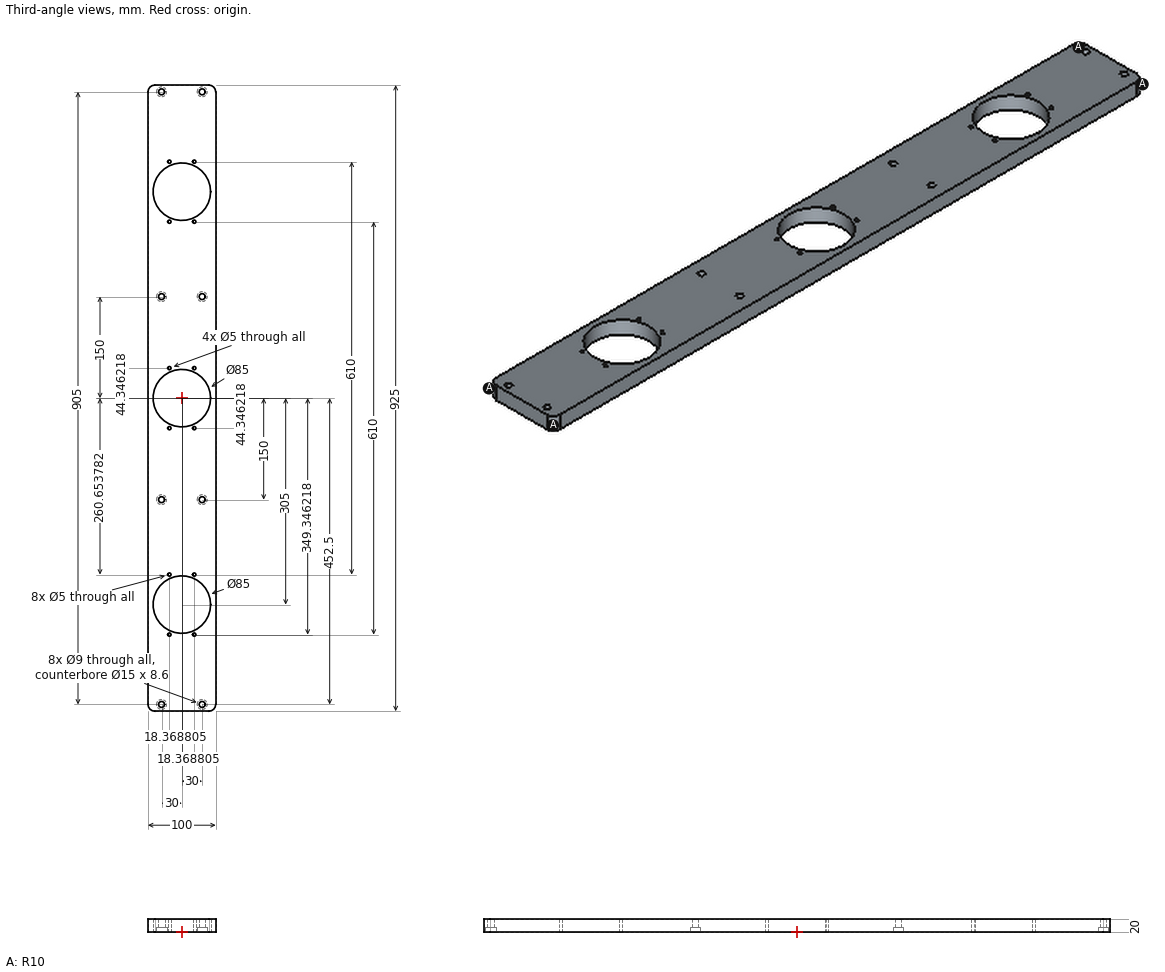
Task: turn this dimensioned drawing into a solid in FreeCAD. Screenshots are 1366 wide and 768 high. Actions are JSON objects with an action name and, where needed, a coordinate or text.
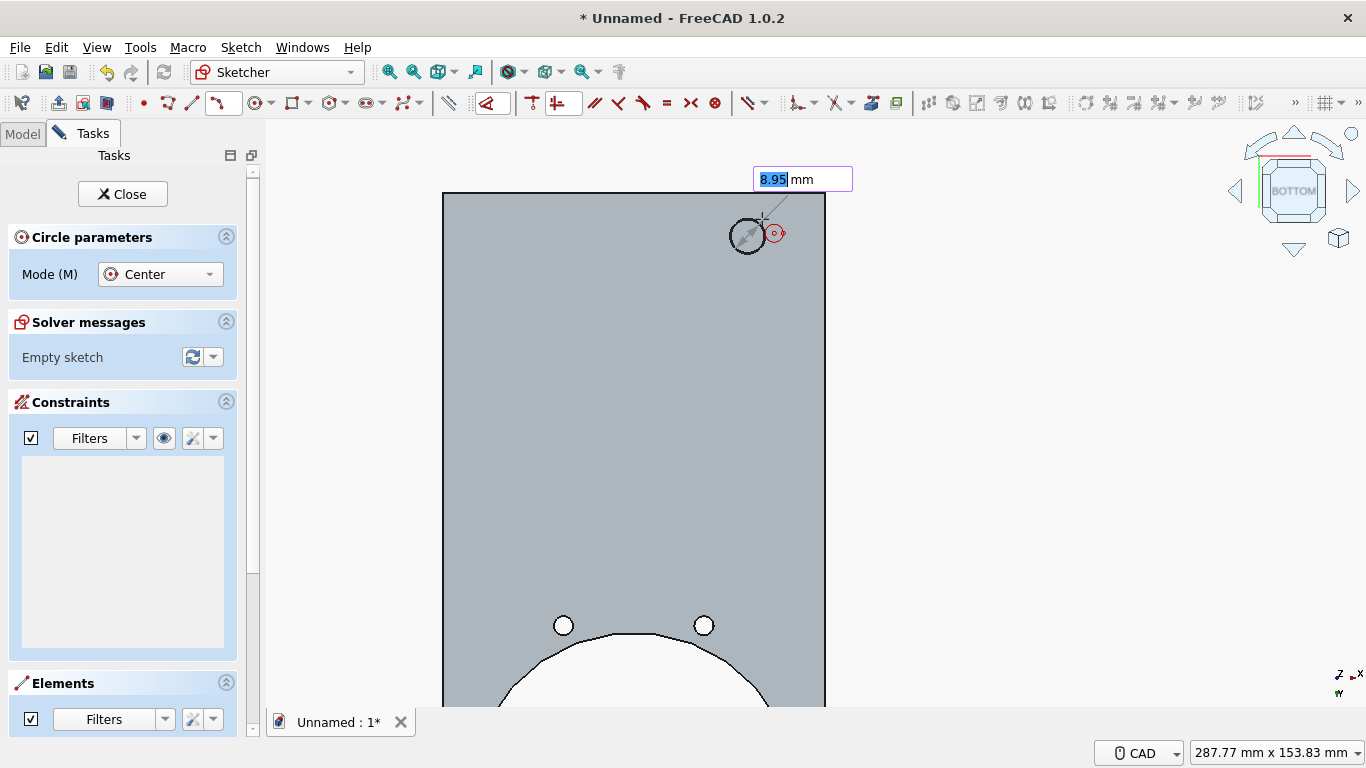
{"action": "left_click", "coordinate": [761, 219]}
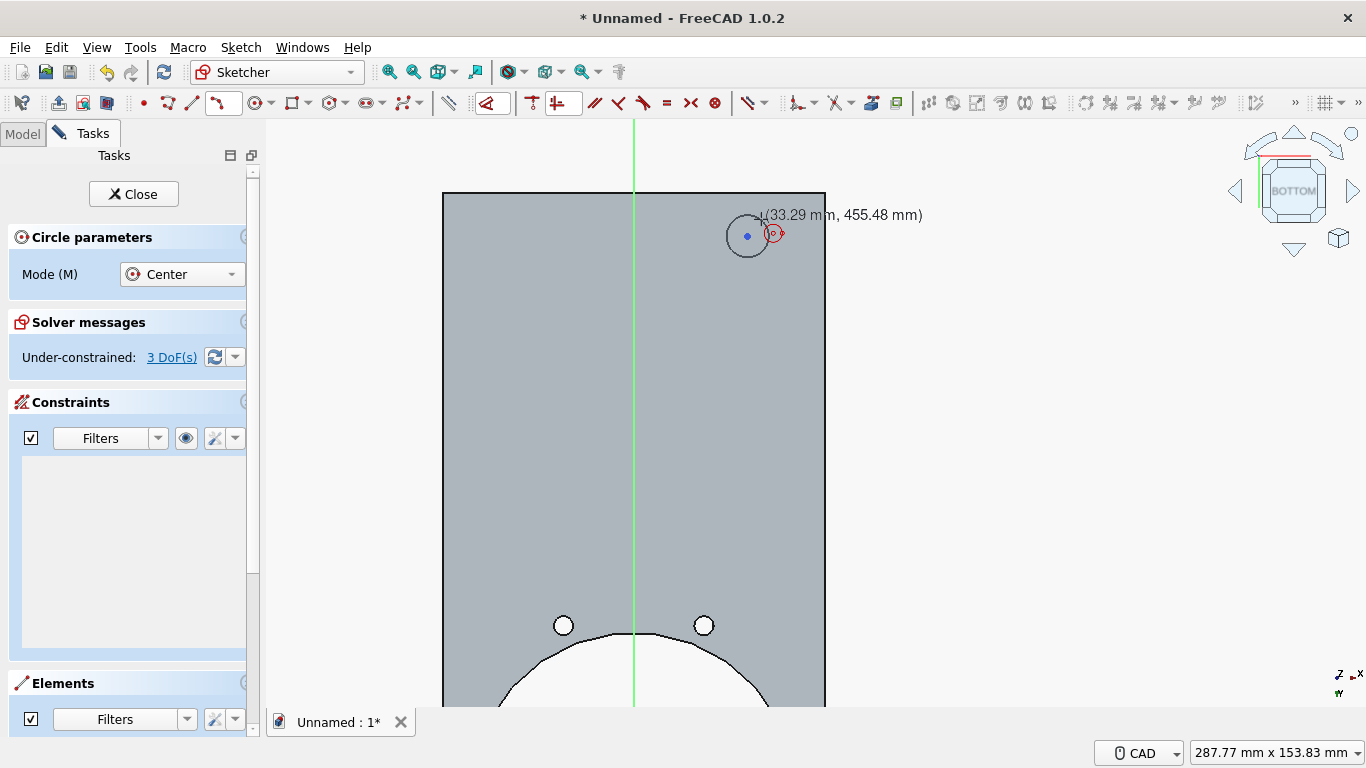
{"action": "scroll", "coordinate": [519, 231], "scroll_direction": "up", "scroll_amount": 2}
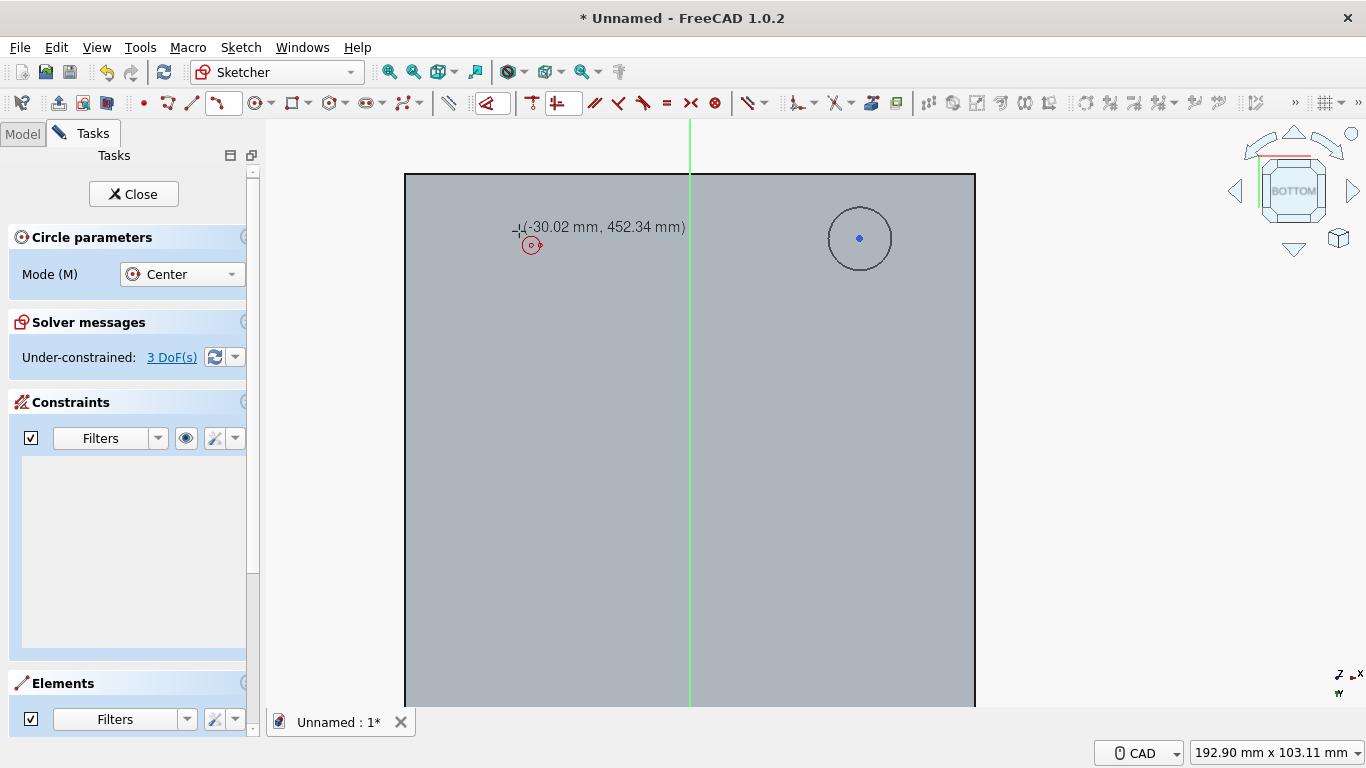
{"action": "scroll", "coordinate": [752, 221], "scroll_direction": "down", "scroll_amount": 13}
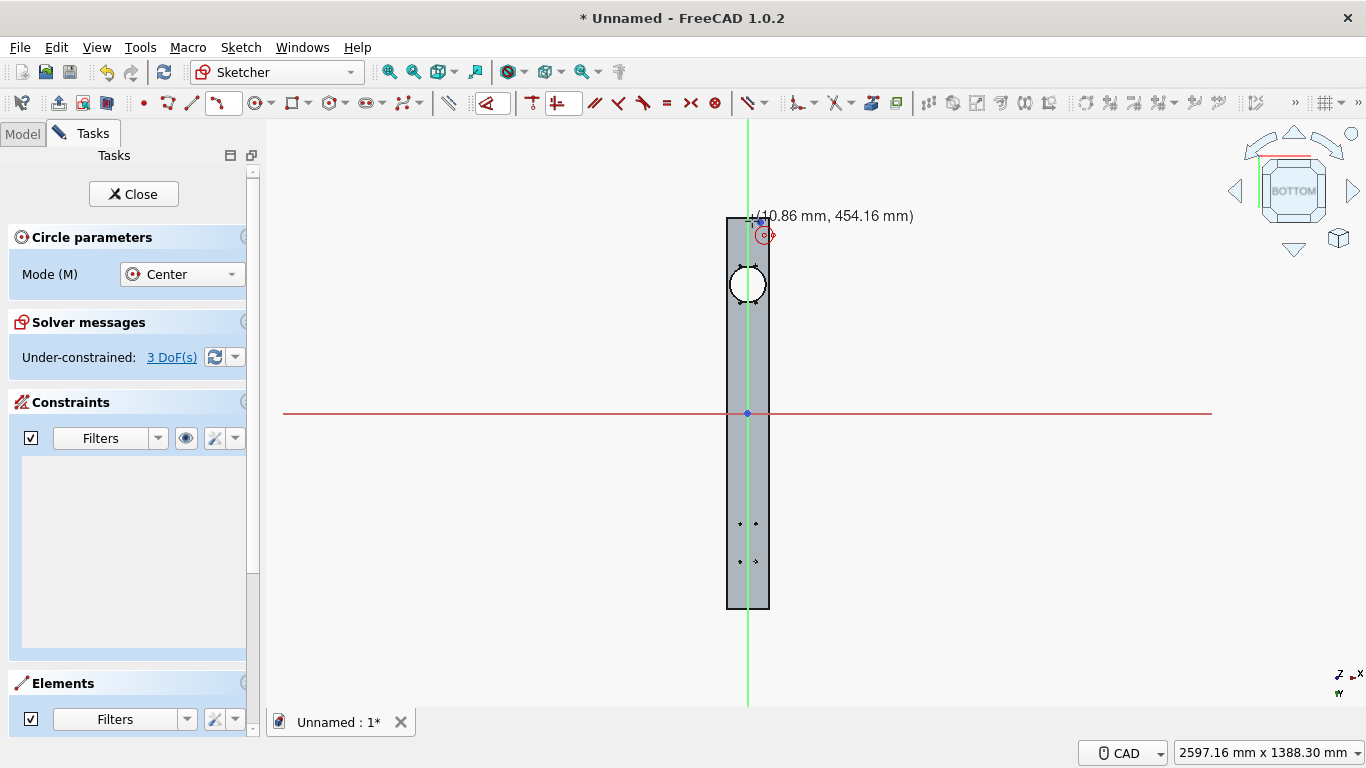
{"action": "scroll", "coordinate": [735, 222], "scroll_direction": "up", "scroll_amount": 2}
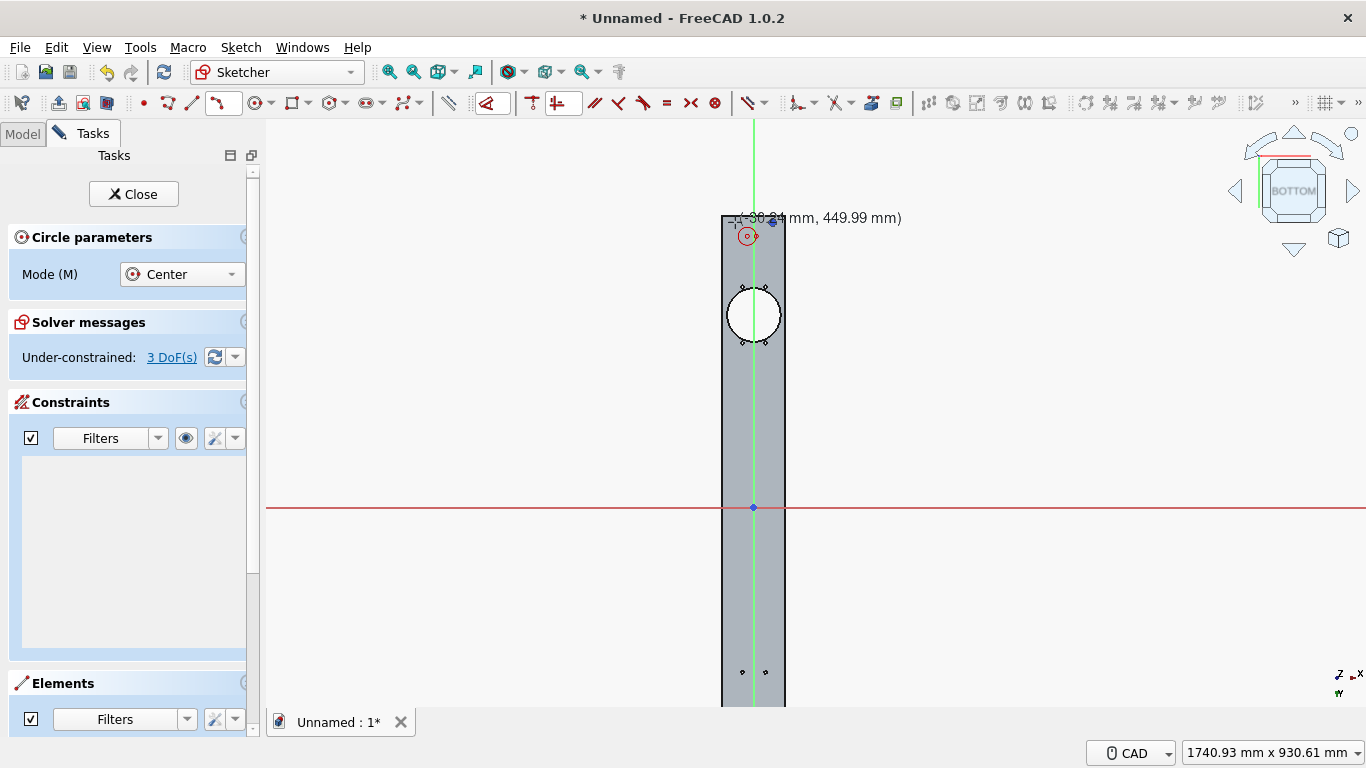
{"action": "left_click", "coordinate": [735, 222]}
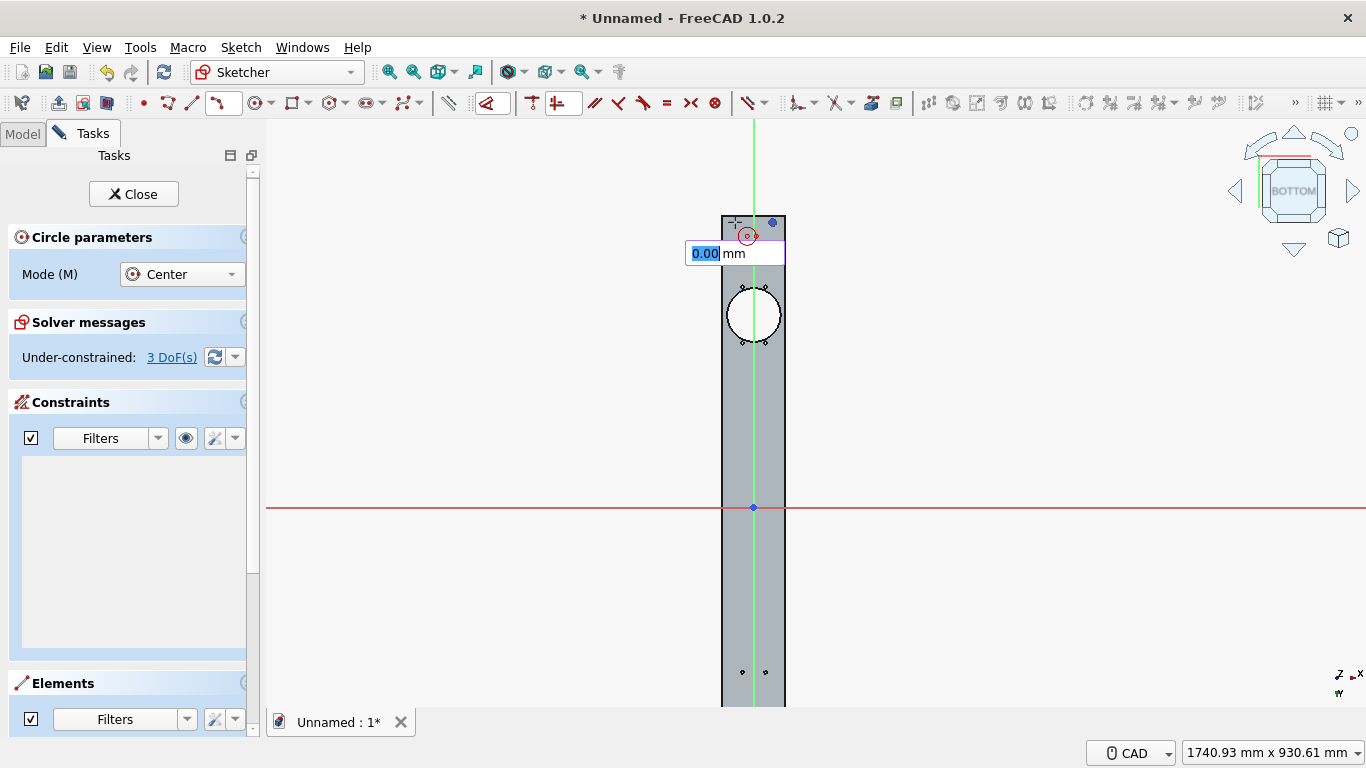
{"action": "scroll", "coordinate": [737, 220], "scroll_direction": "up", "scroll_amount": 9}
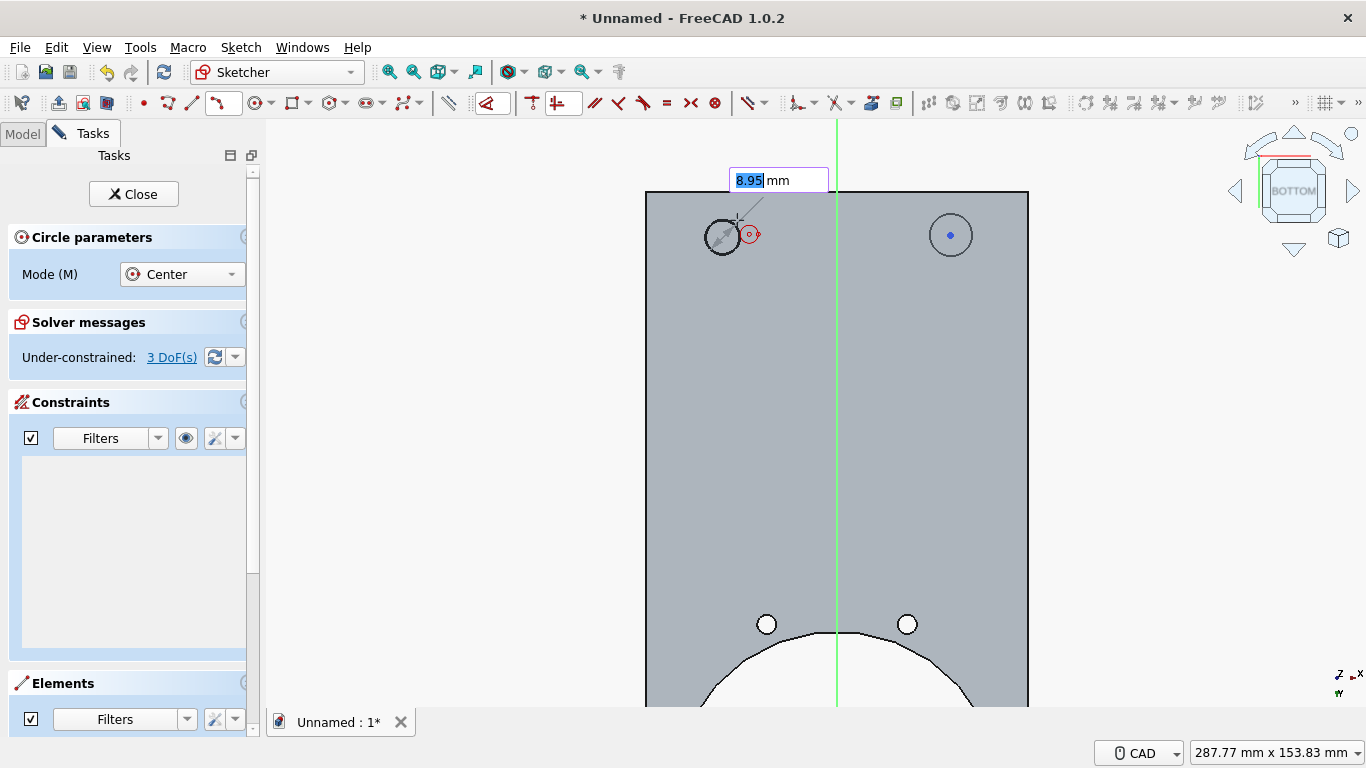
{"action": "left_click", "coordinate": [735, 218]}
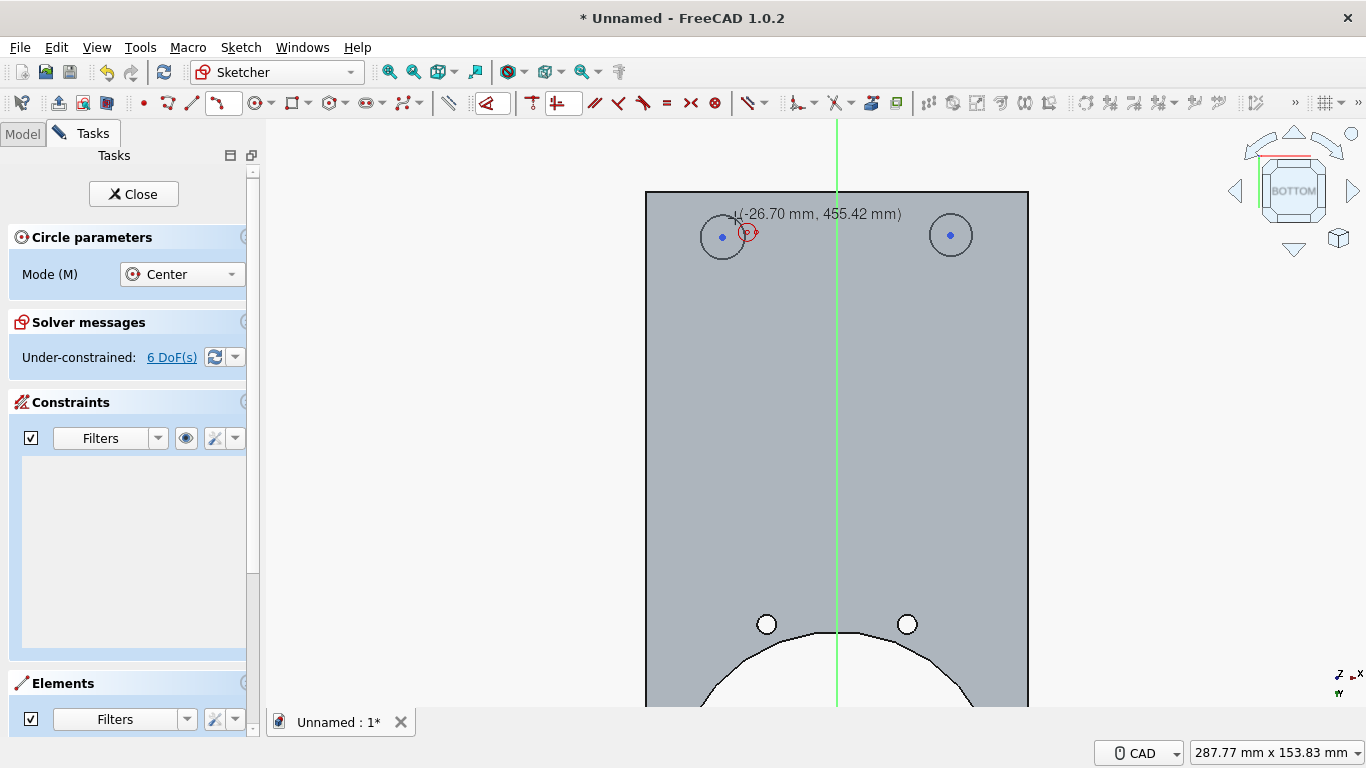
{"action": "scroll", "coordinate": [736, 220], "scroll_direction": "down", "scroll_amount": 11}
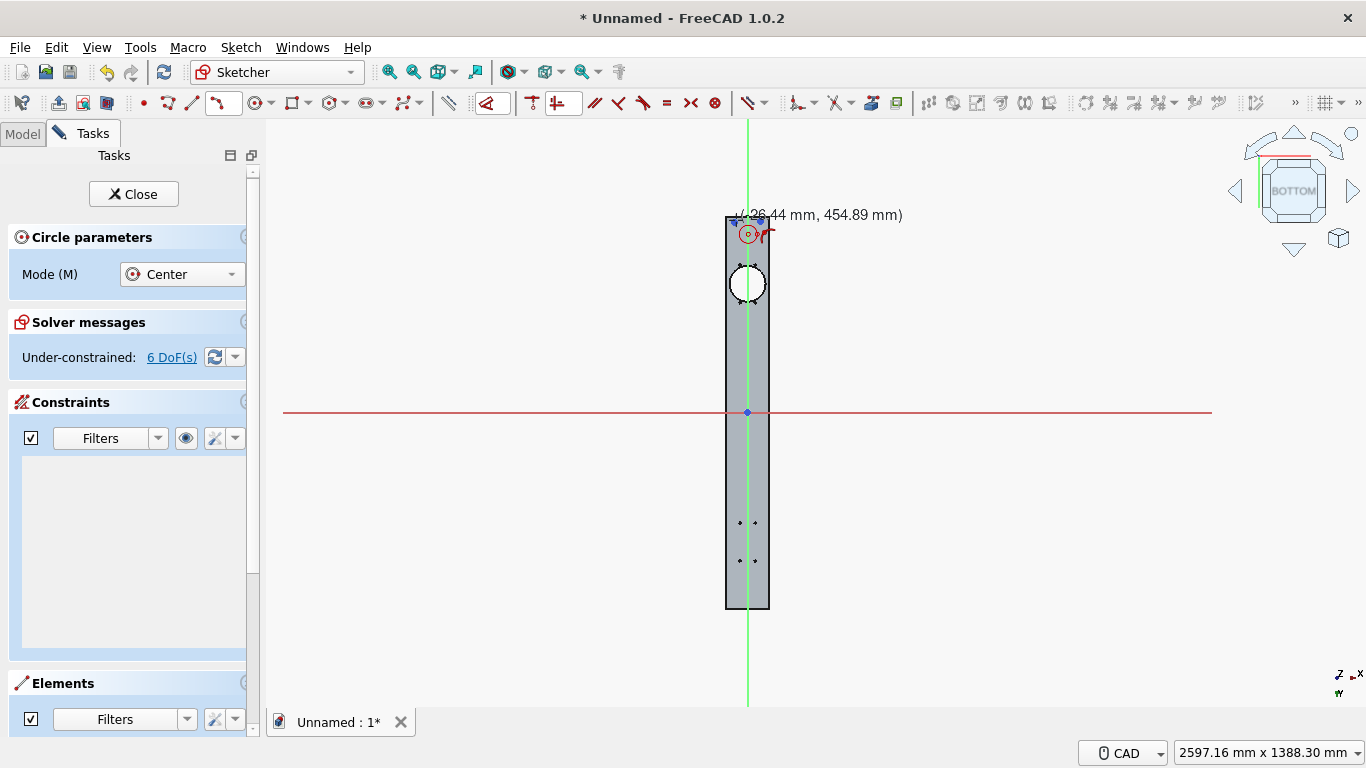
{"action": "scroll", "coordinate": [760, 349], "scroll_direction": "up", "scroll_amount": 13}